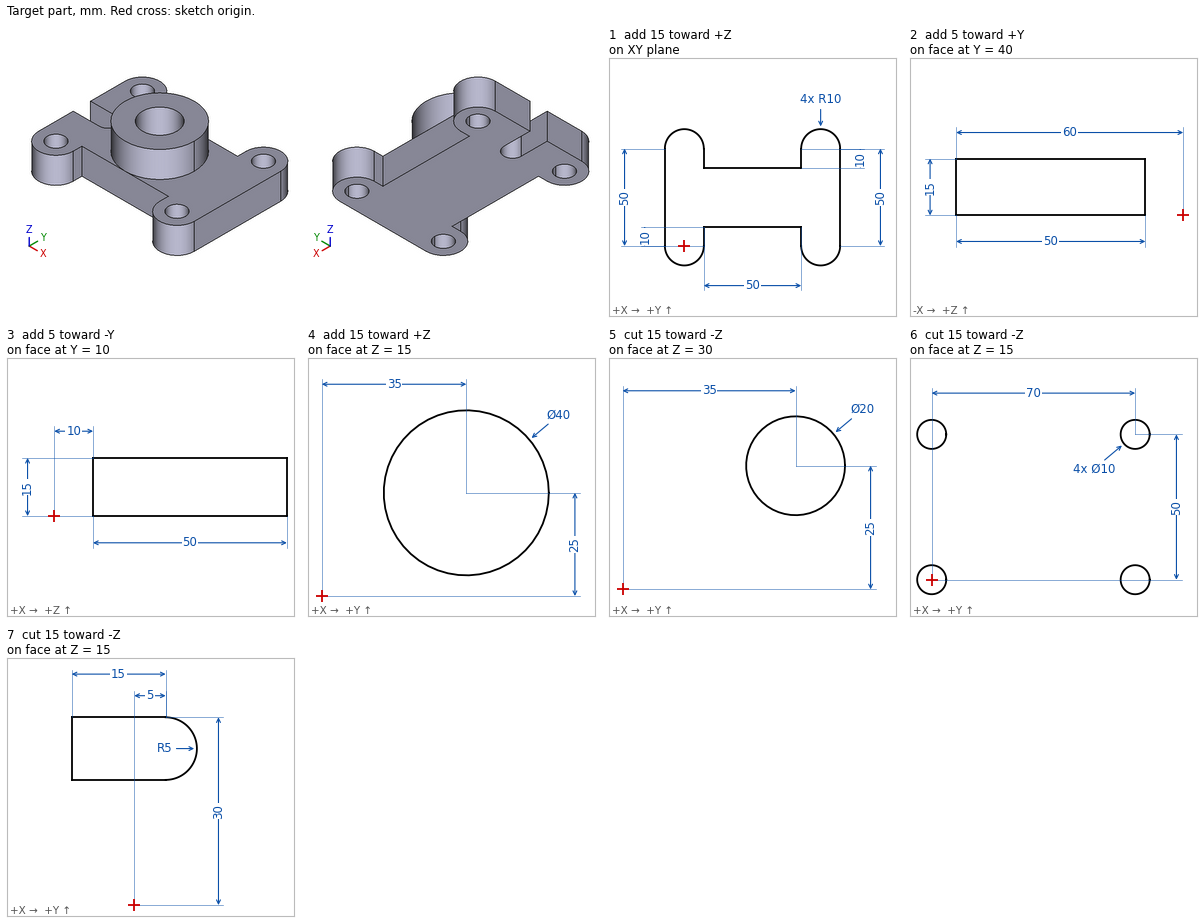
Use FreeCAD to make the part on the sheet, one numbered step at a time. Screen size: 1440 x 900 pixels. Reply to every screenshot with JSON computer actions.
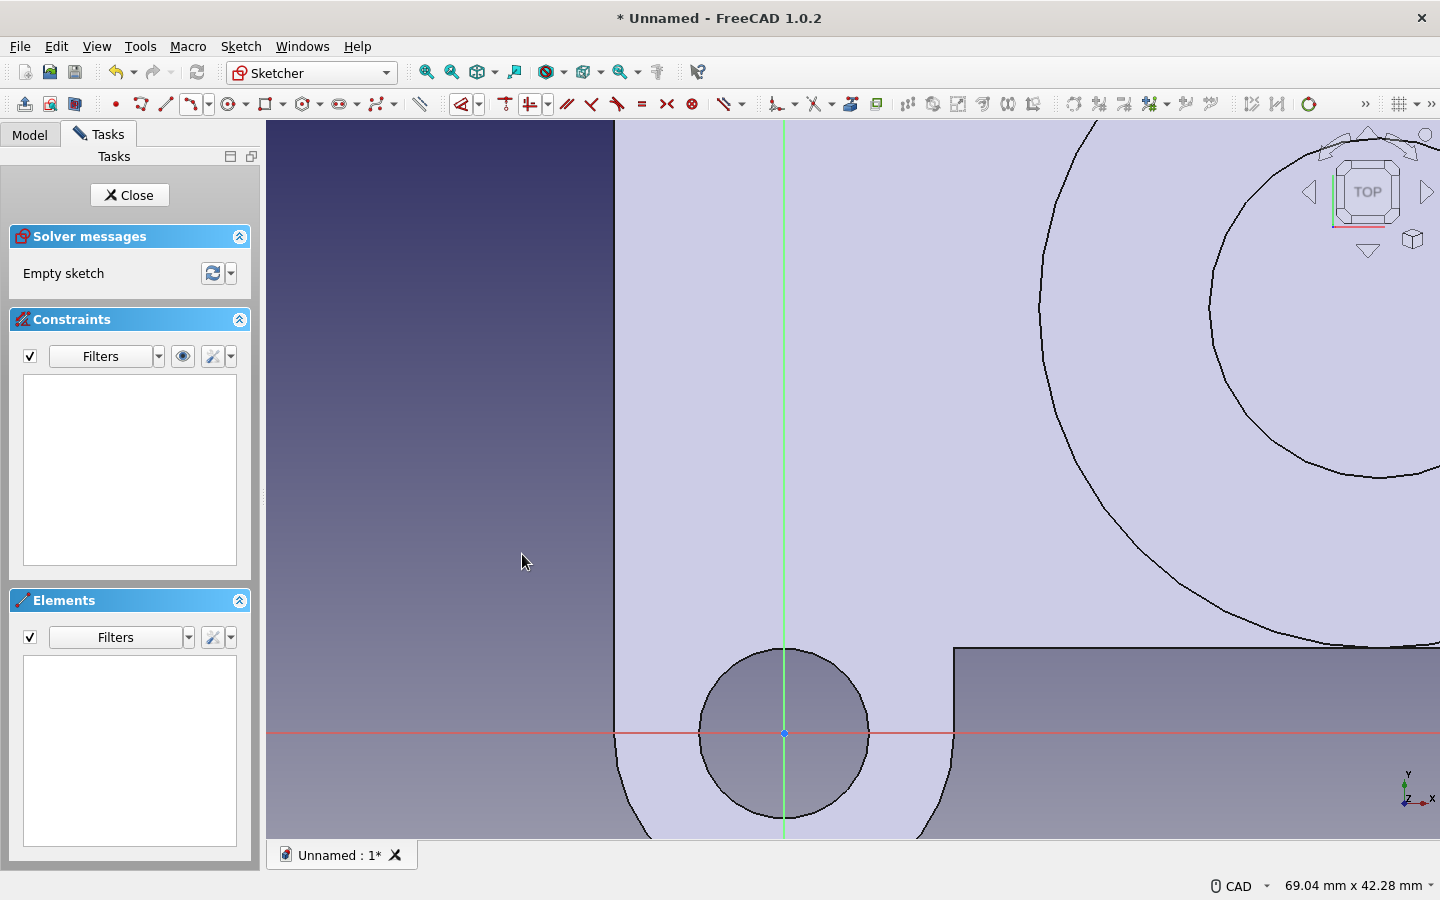
{"action": "key", "text": "g m"}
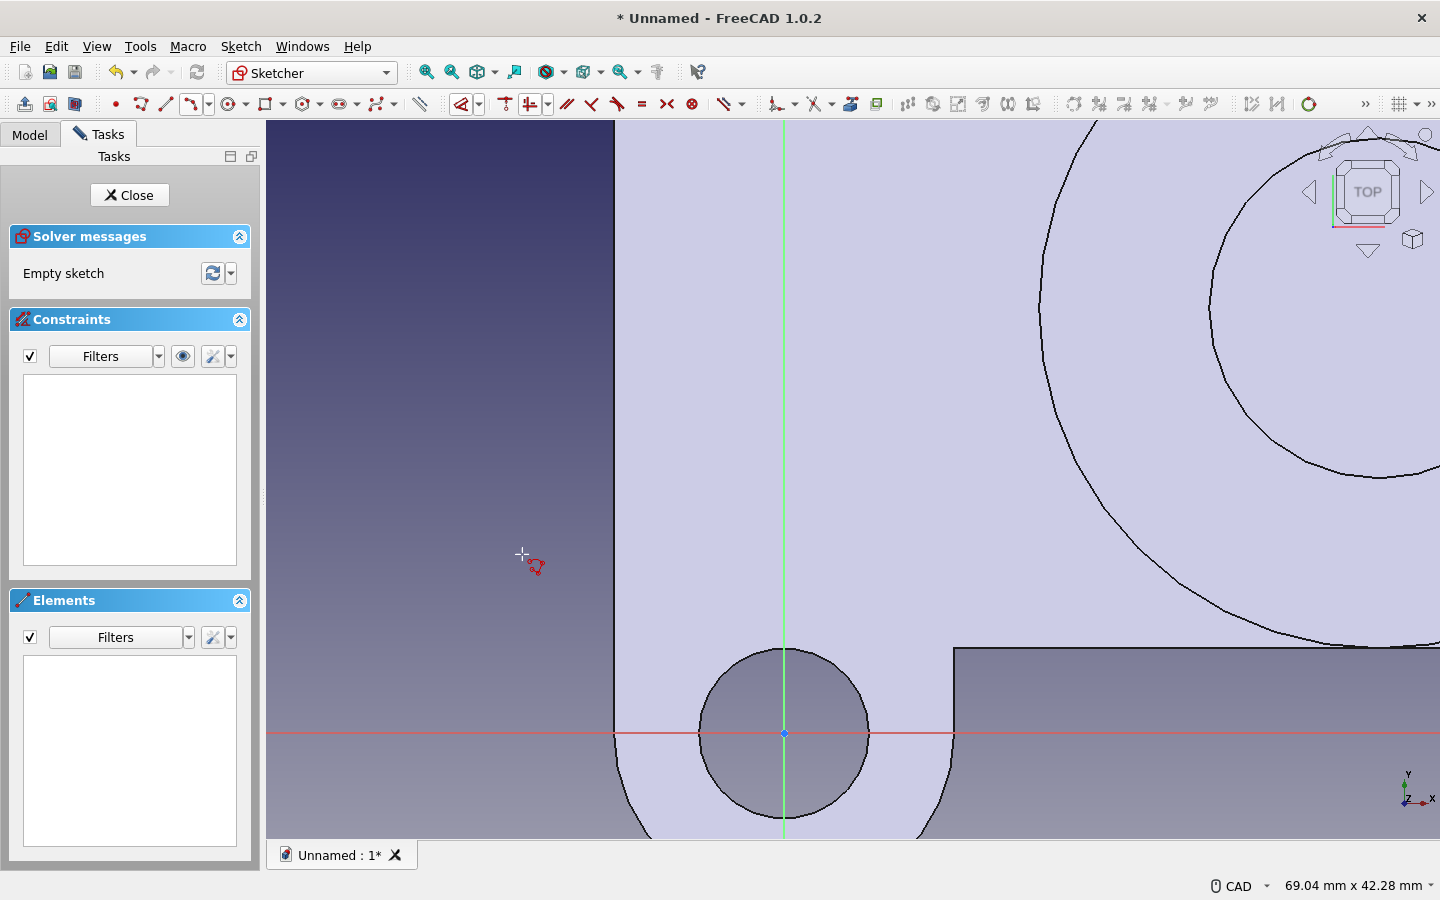
{"action": "left_click", "coordinate": [869, 223]}
{"action": "left_click", "coordinate": [614, 223]}
{"action": "left_click", "coordinate": [614, 393]}
{"action": "left_click", "coordinate": [869, 393]}
{"action": "right_click", "coordinate": [869, 393]}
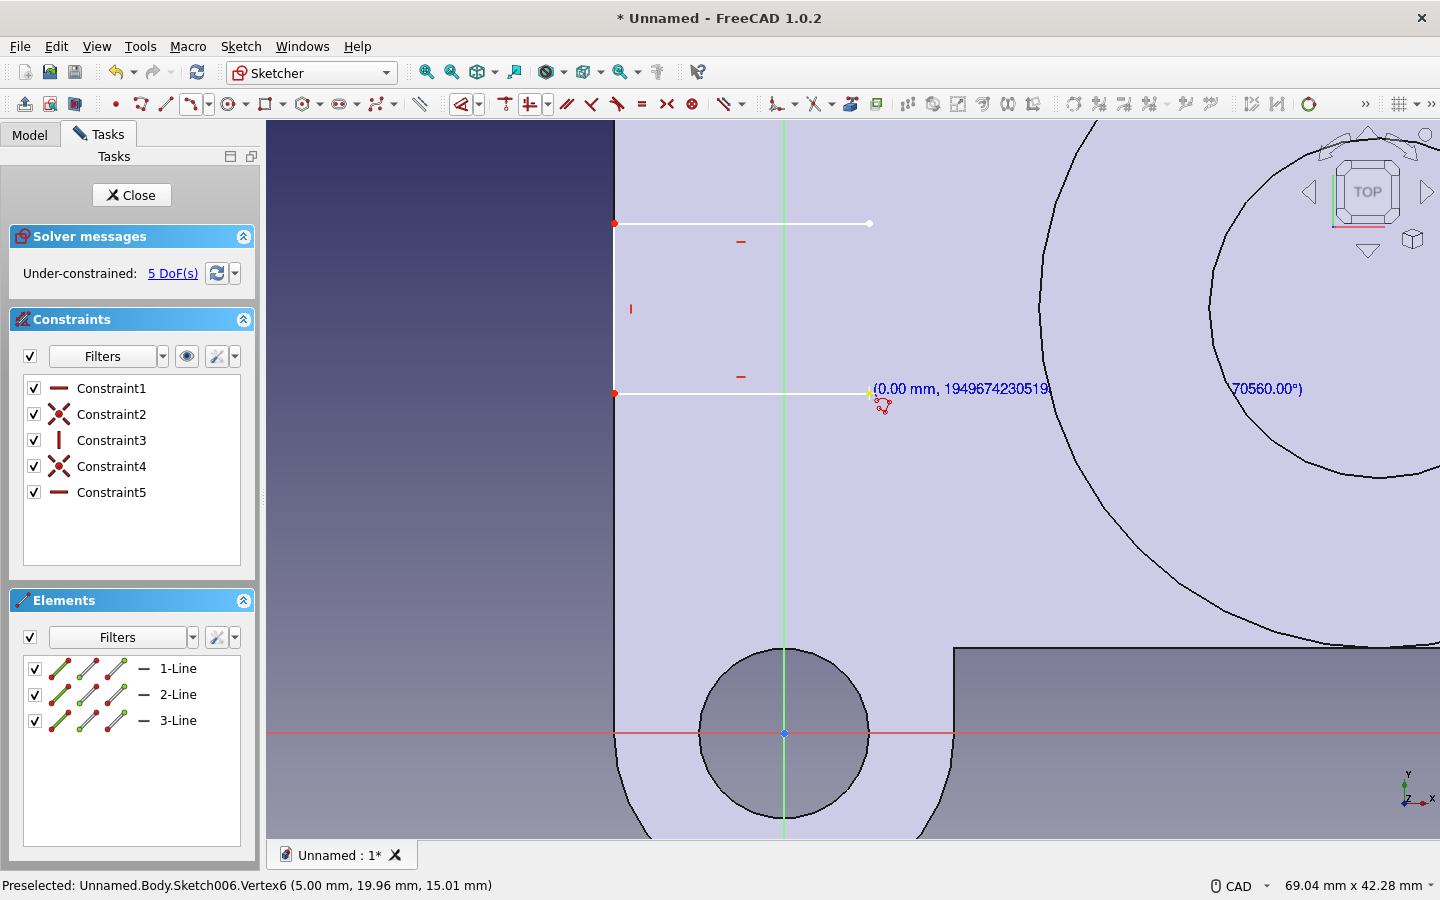
{"action": "key", "text": "g 3 a"}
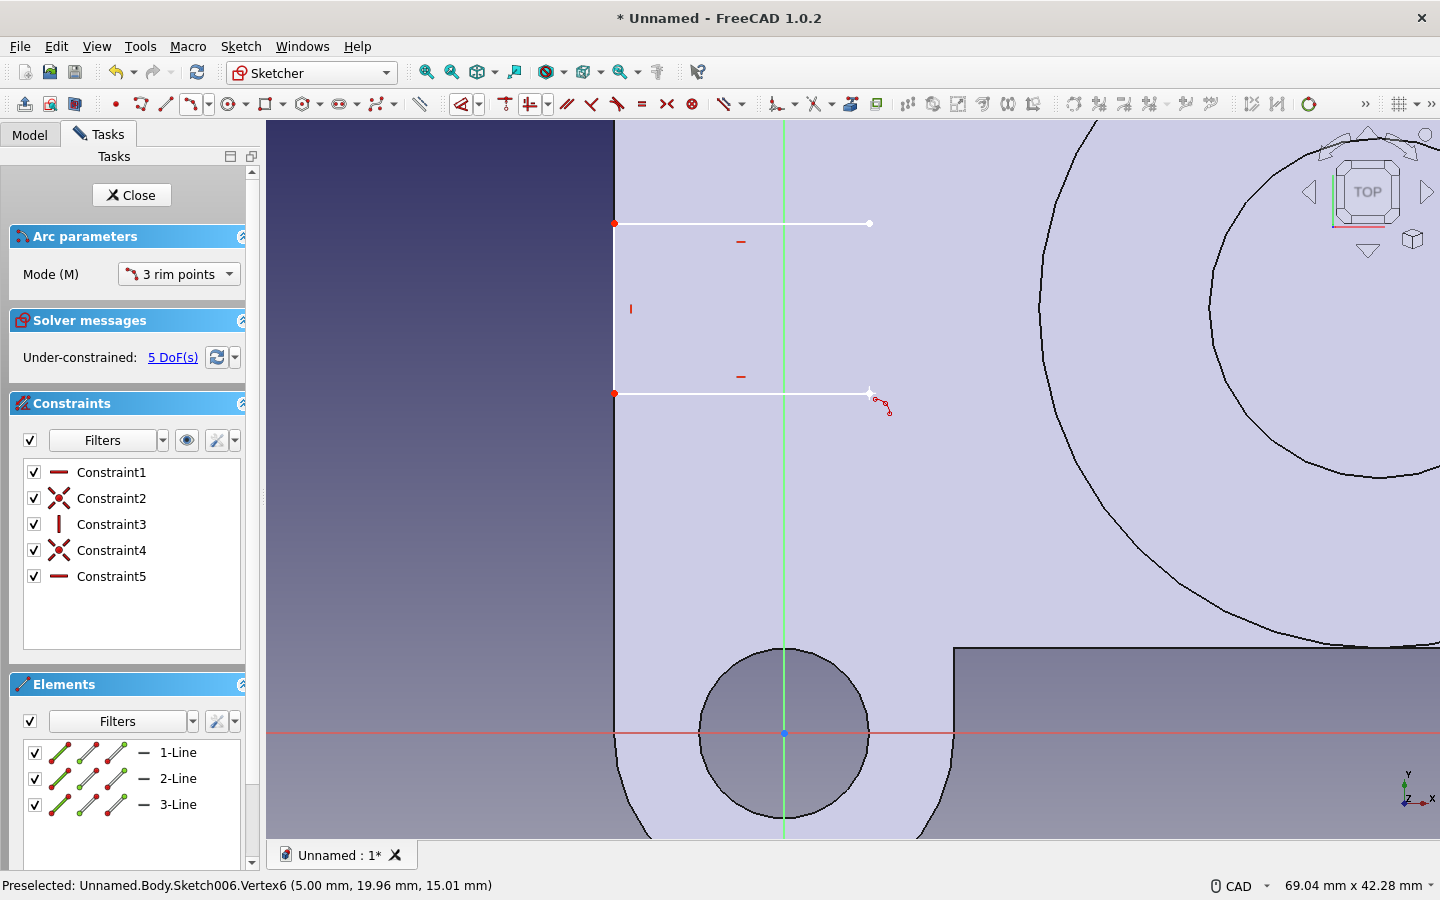
{"action": "left_click", "coordinate": [869, 394]}
{"action": "left_click", "coordinate": [869, 224]}
{"action": "left_click", "coordinate": [954, 308]}
{"action": "key", "text": "Escape"}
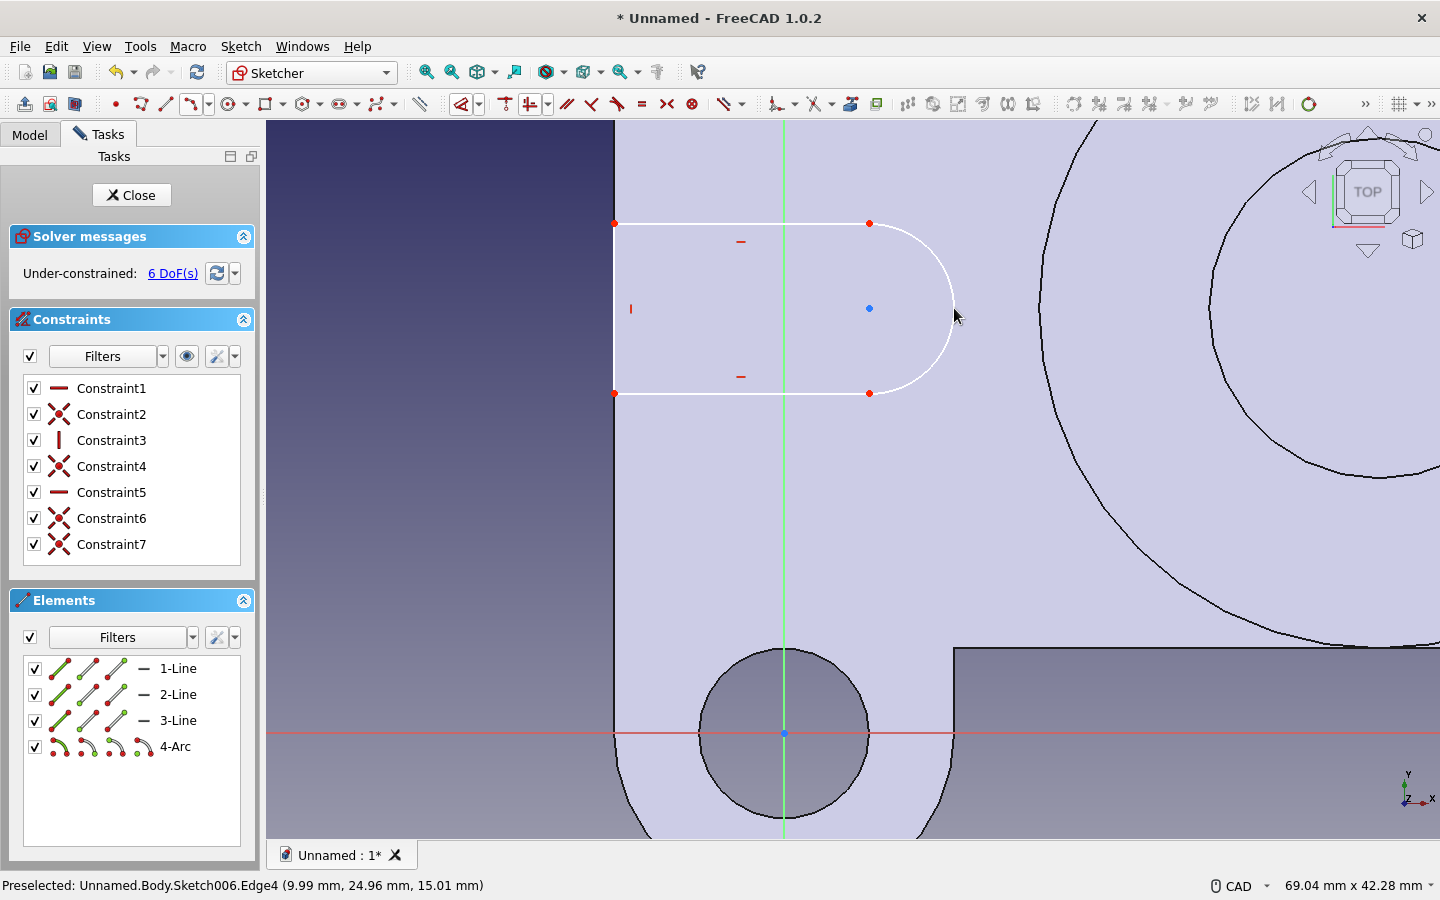
{"action": "left_click", "coordinate": [690, 224]}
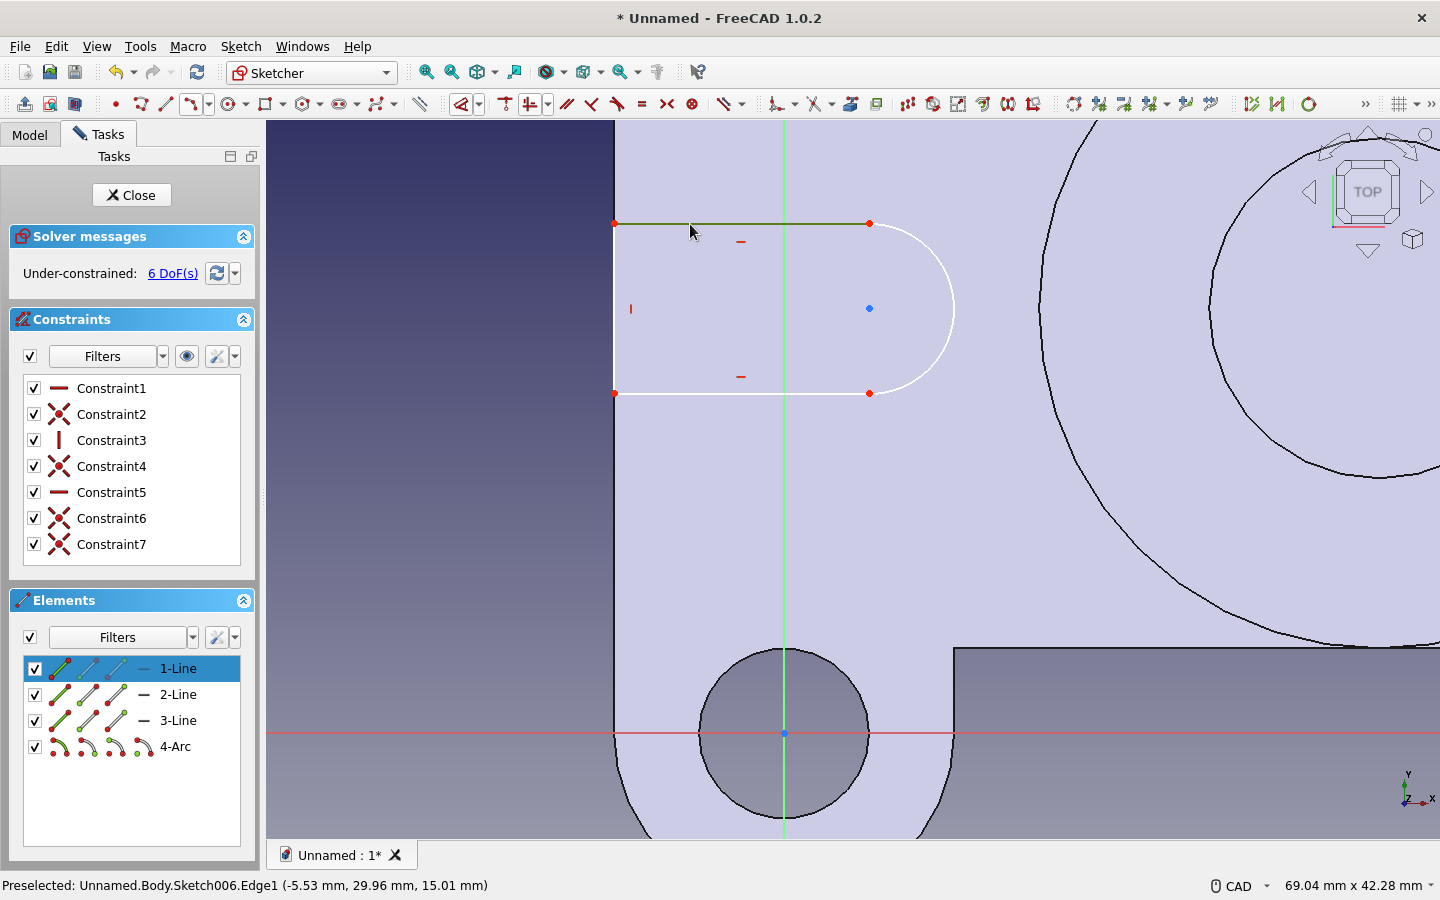
{"action": "left_click", "coordinate": [938, 359]}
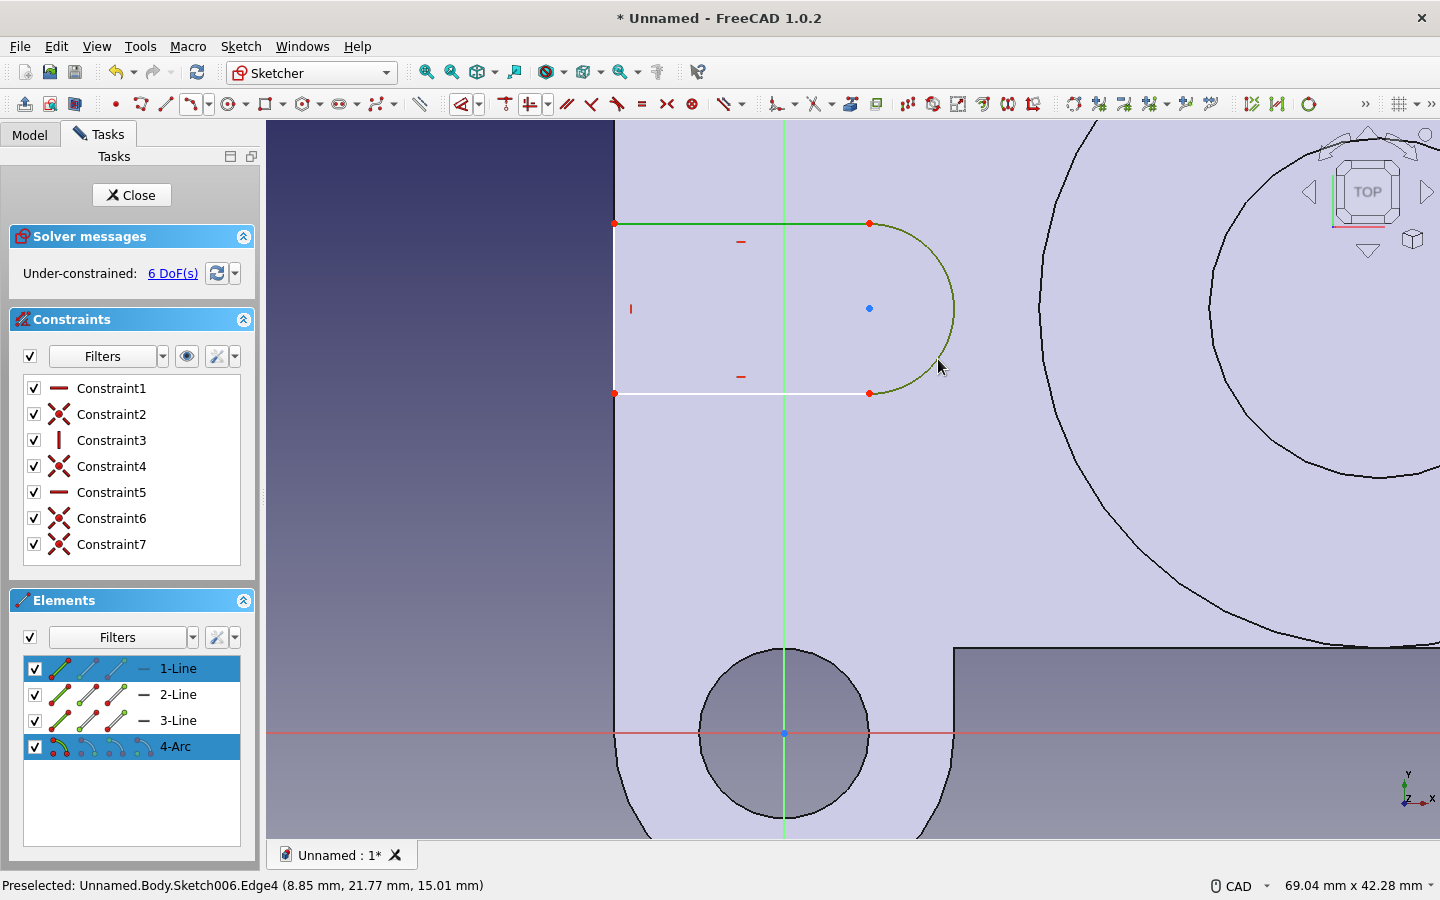
{"action": "left_click", "coordinate": [617, 104]}